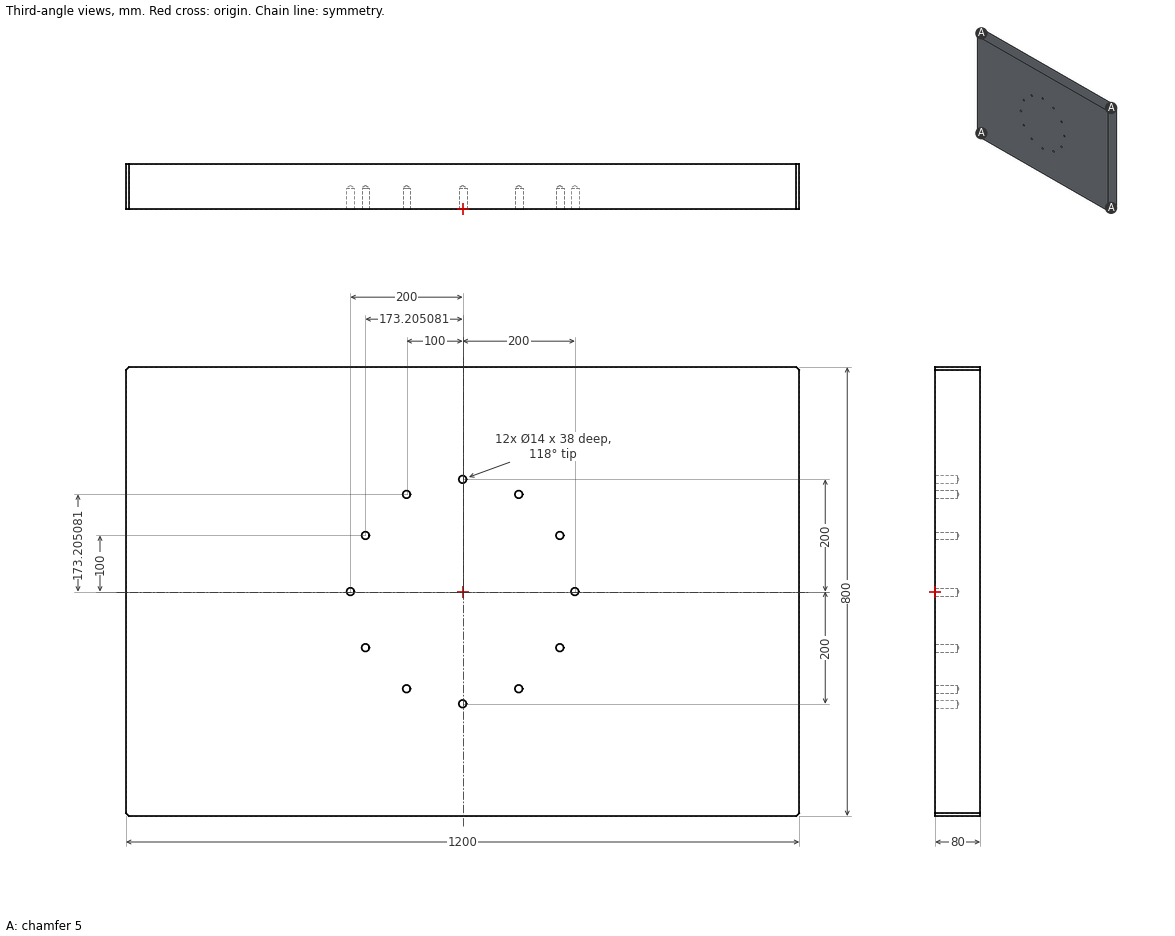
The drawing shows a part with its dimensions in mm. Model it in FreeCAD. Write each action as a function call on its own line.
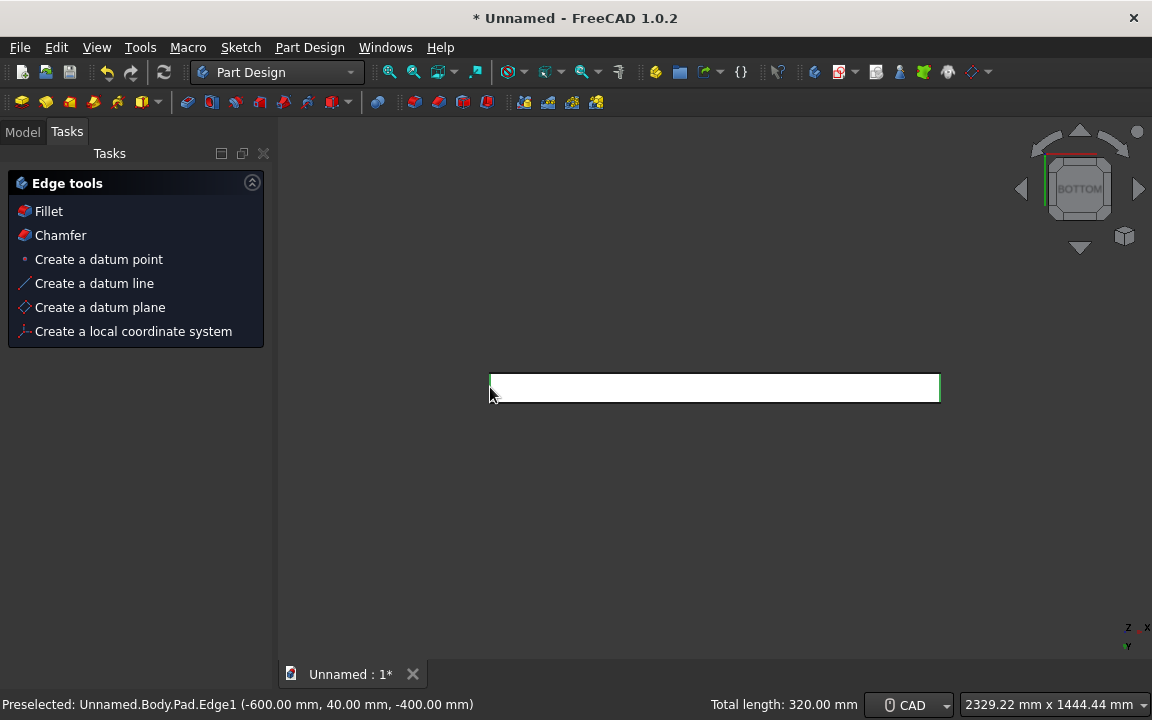
click(440, 102)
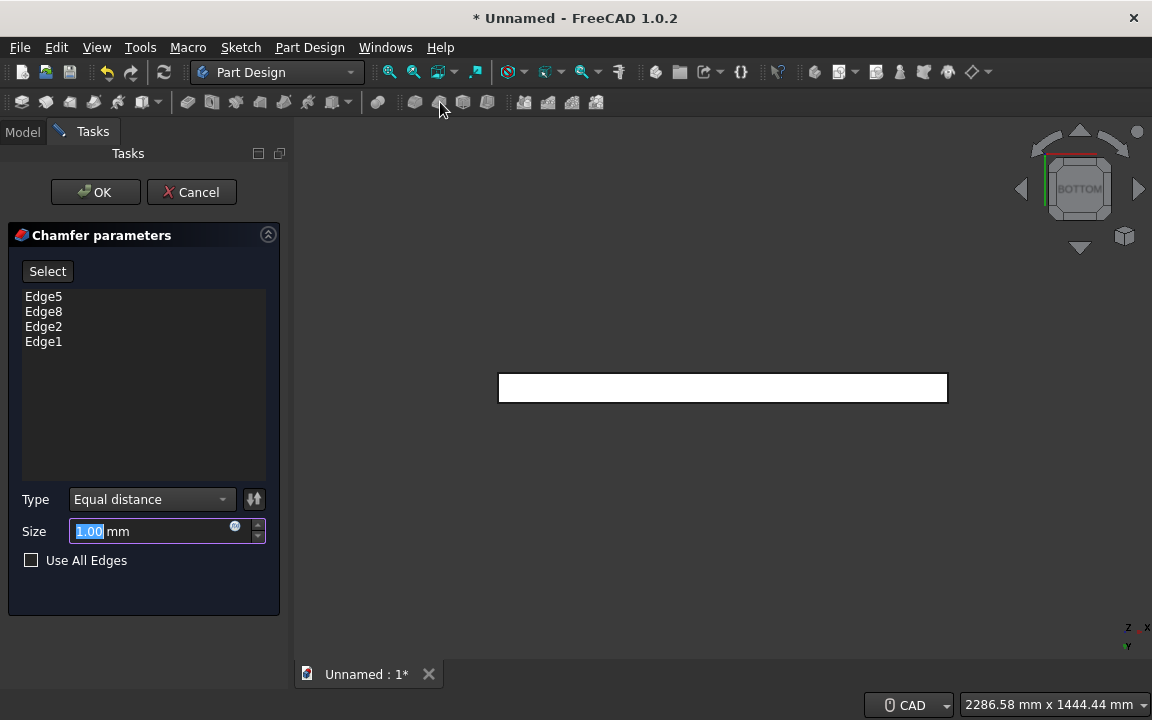
text(5)
key(Tab)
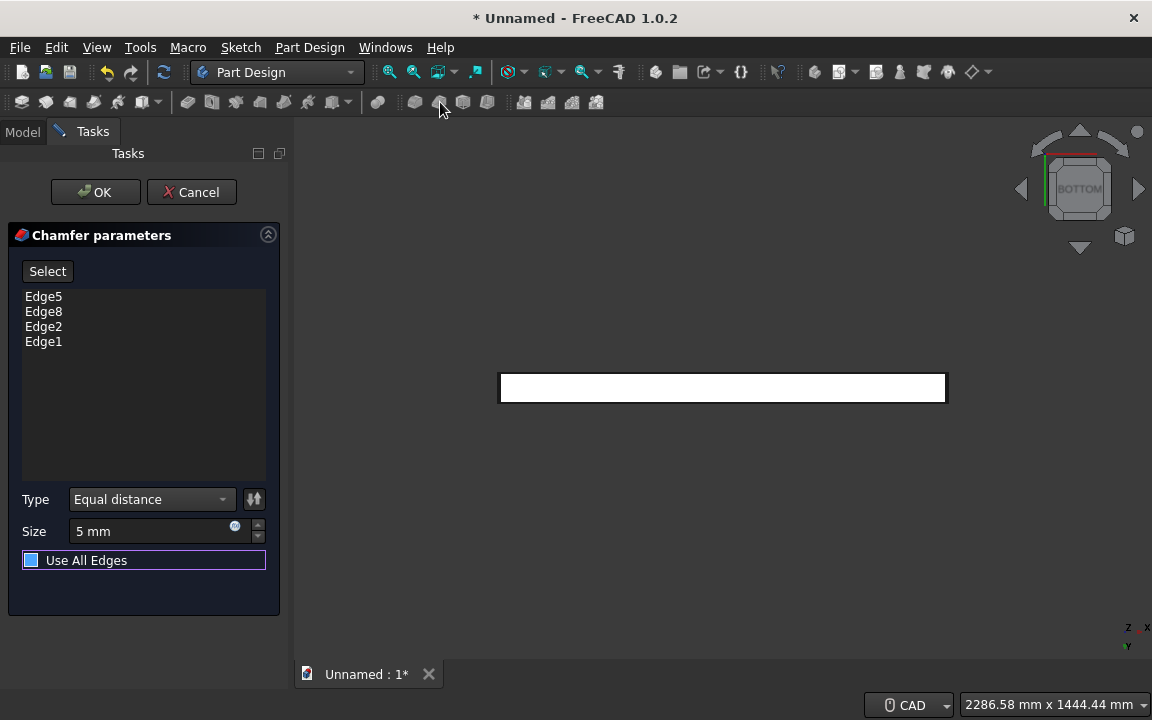
click(96, 192)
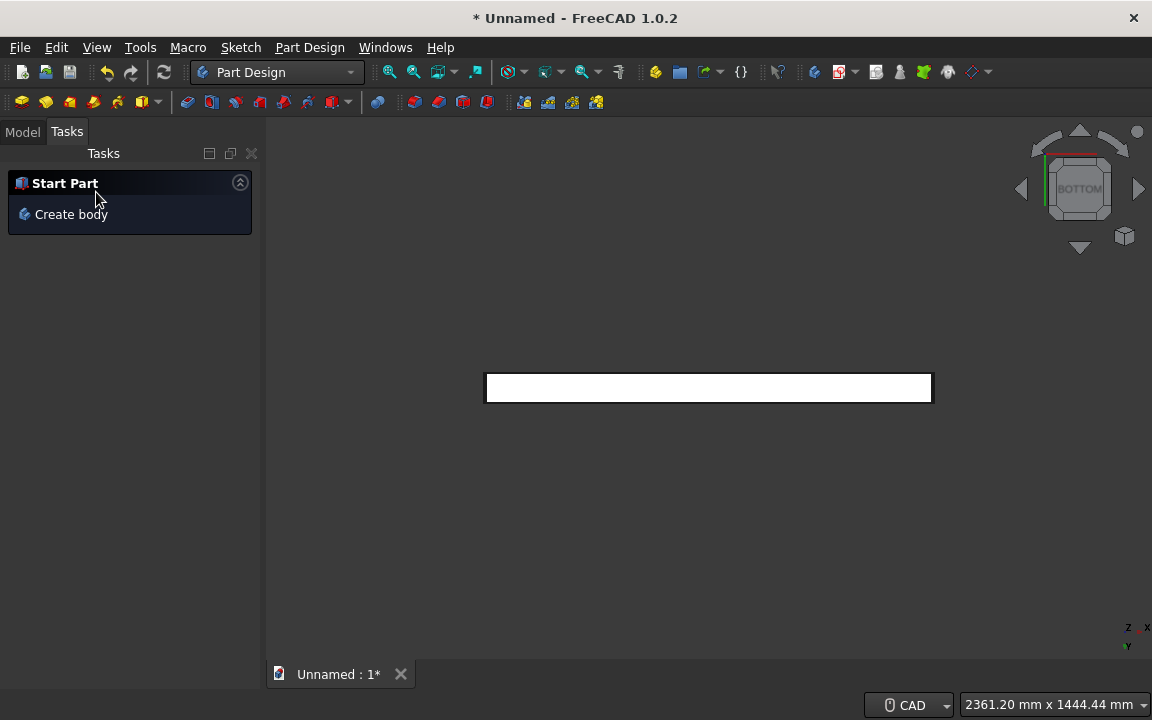
click(840, 72)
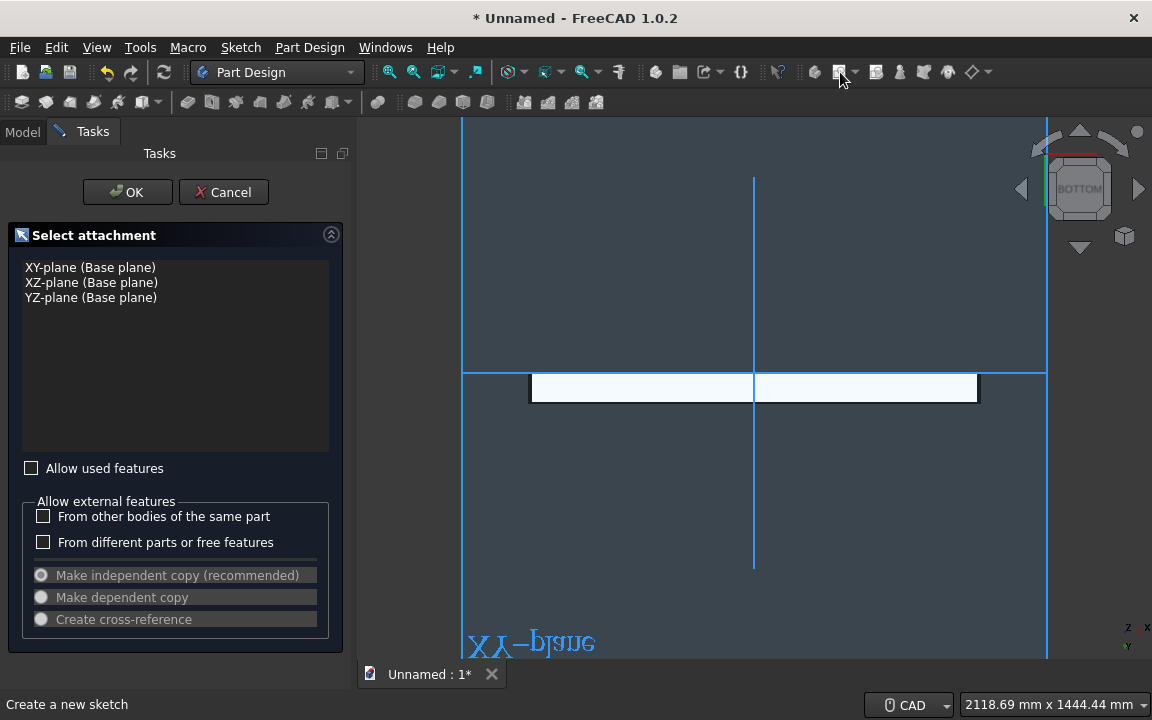
click(82, 282)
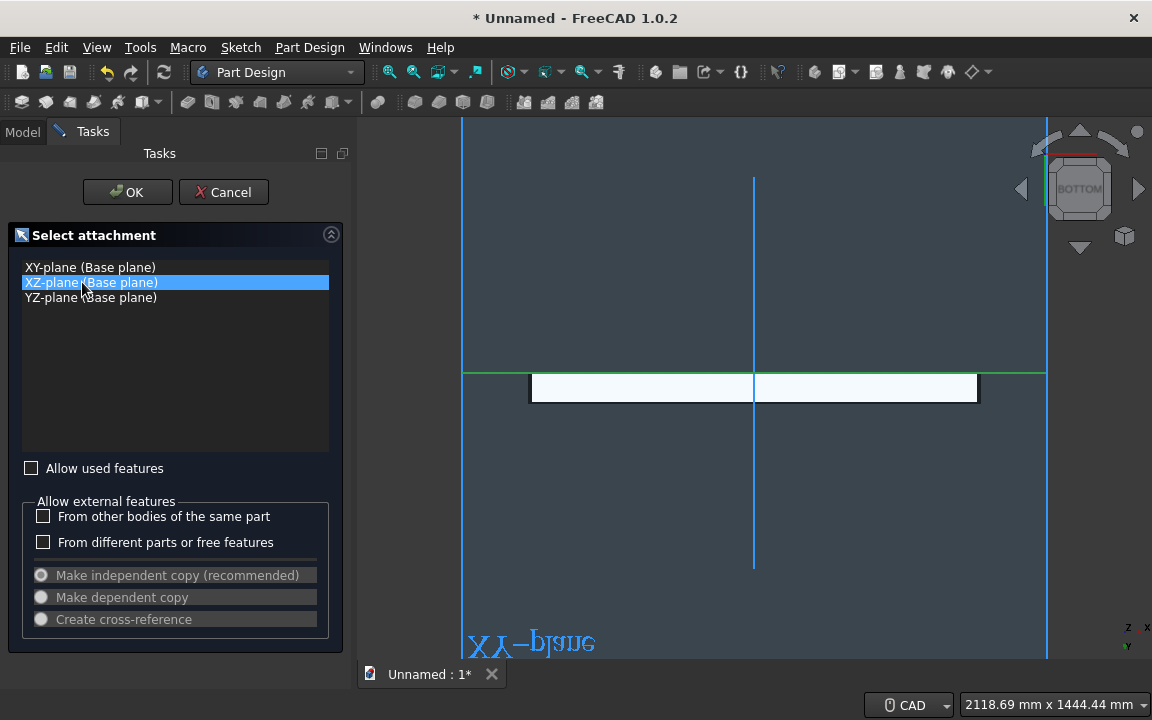
click(128, 192)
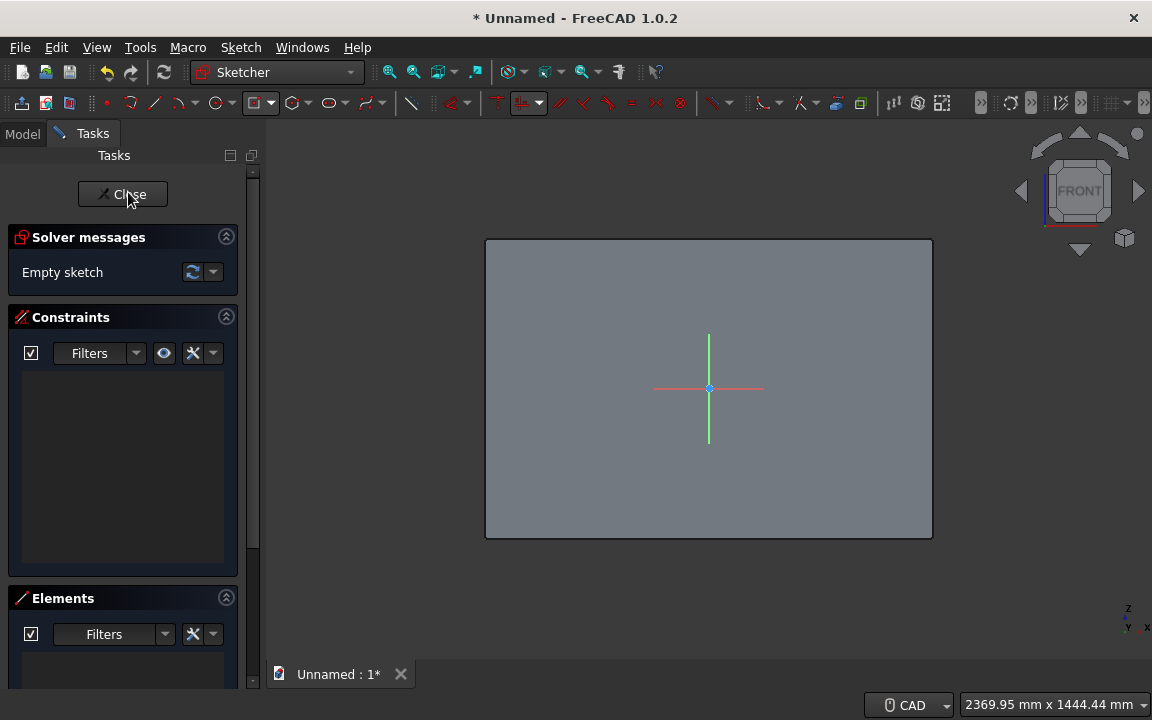
scroll(765, 389, up, 4)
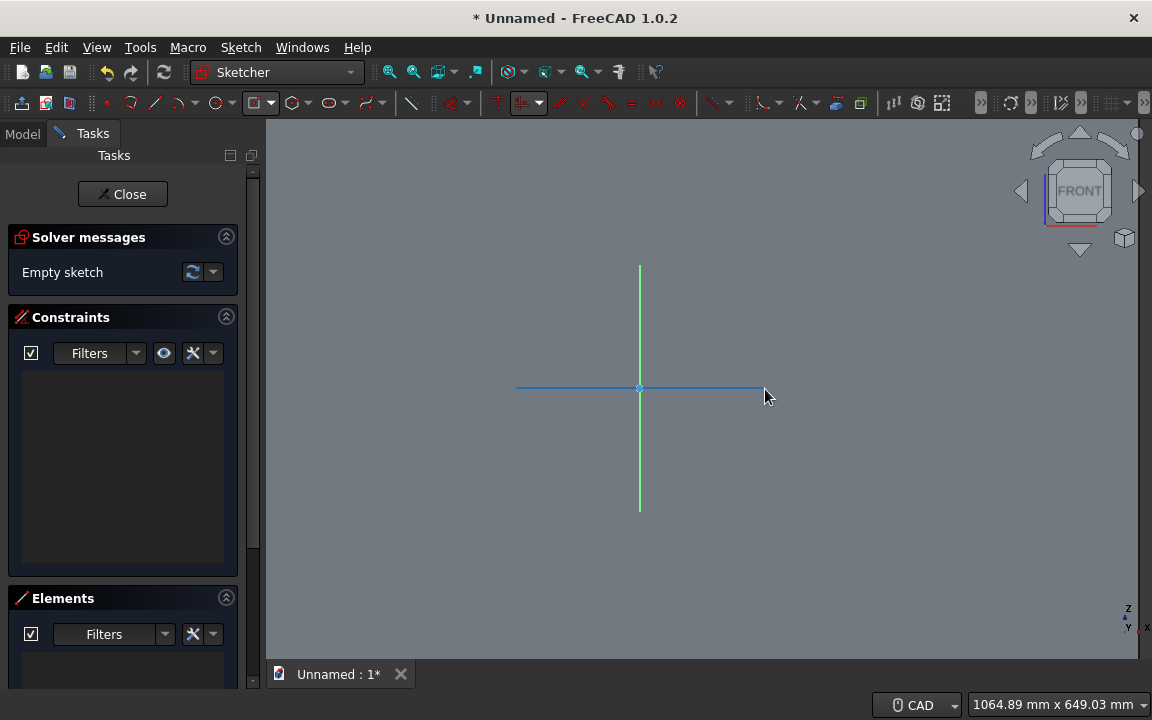
click(216, 104)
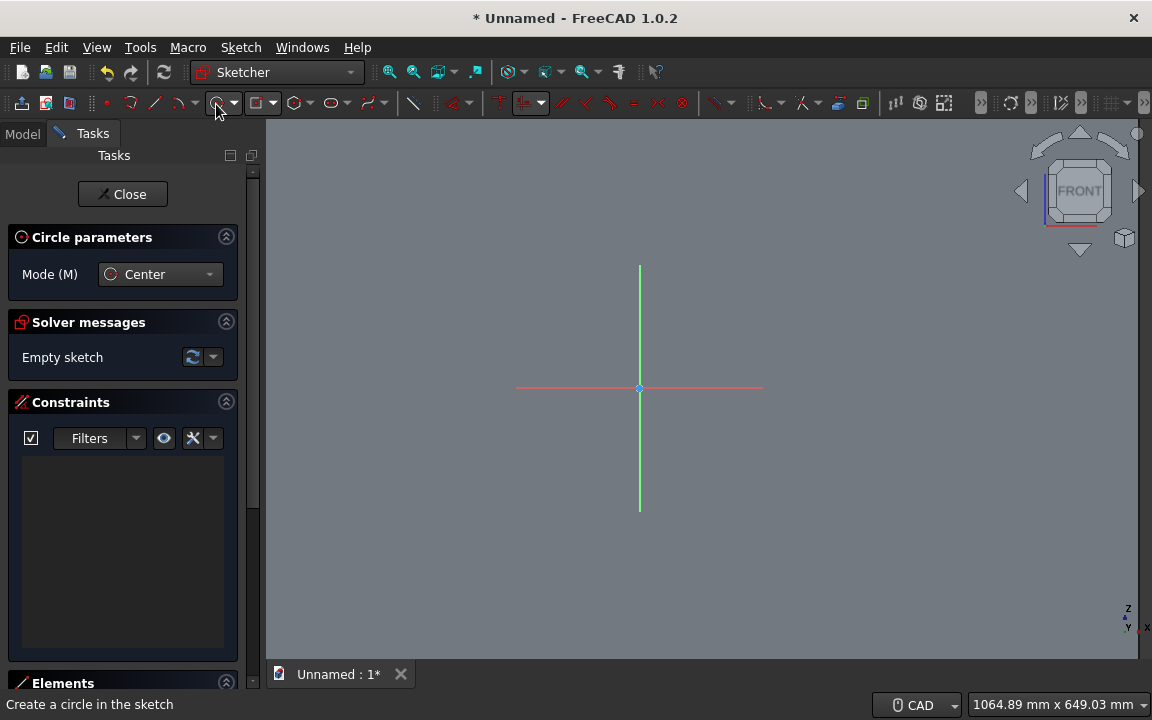
scroll(640, 222, up, 7)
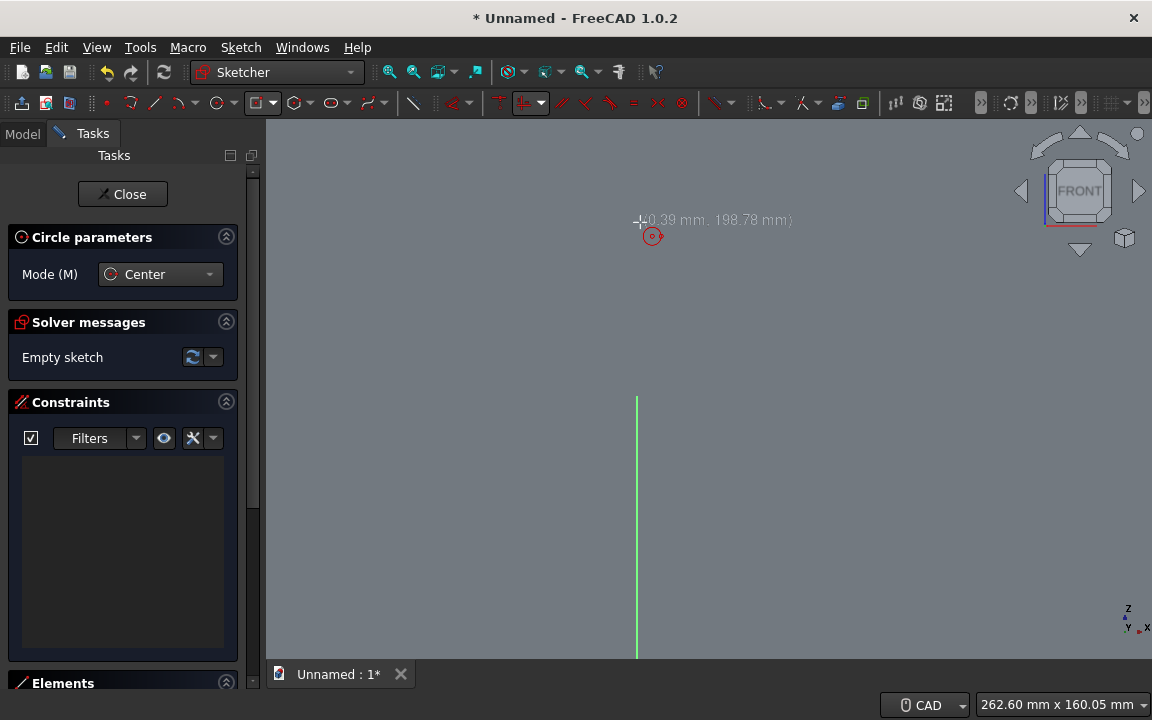
scroll(642, 223, down, 7)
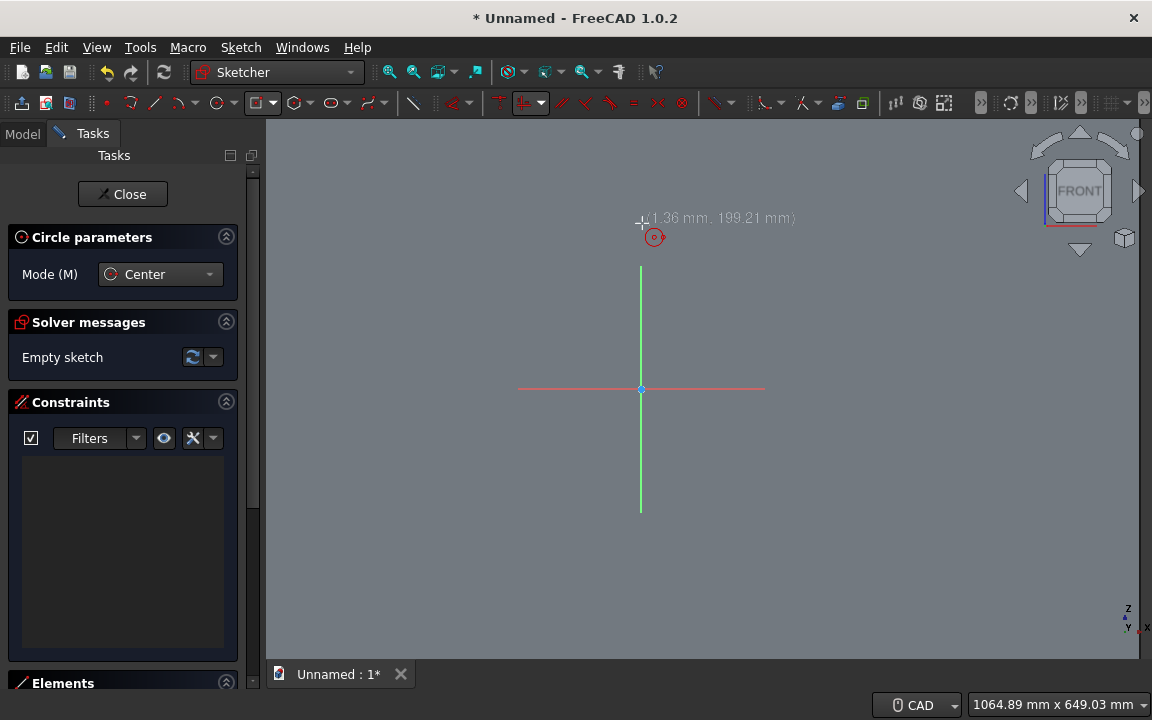
click(641, 223)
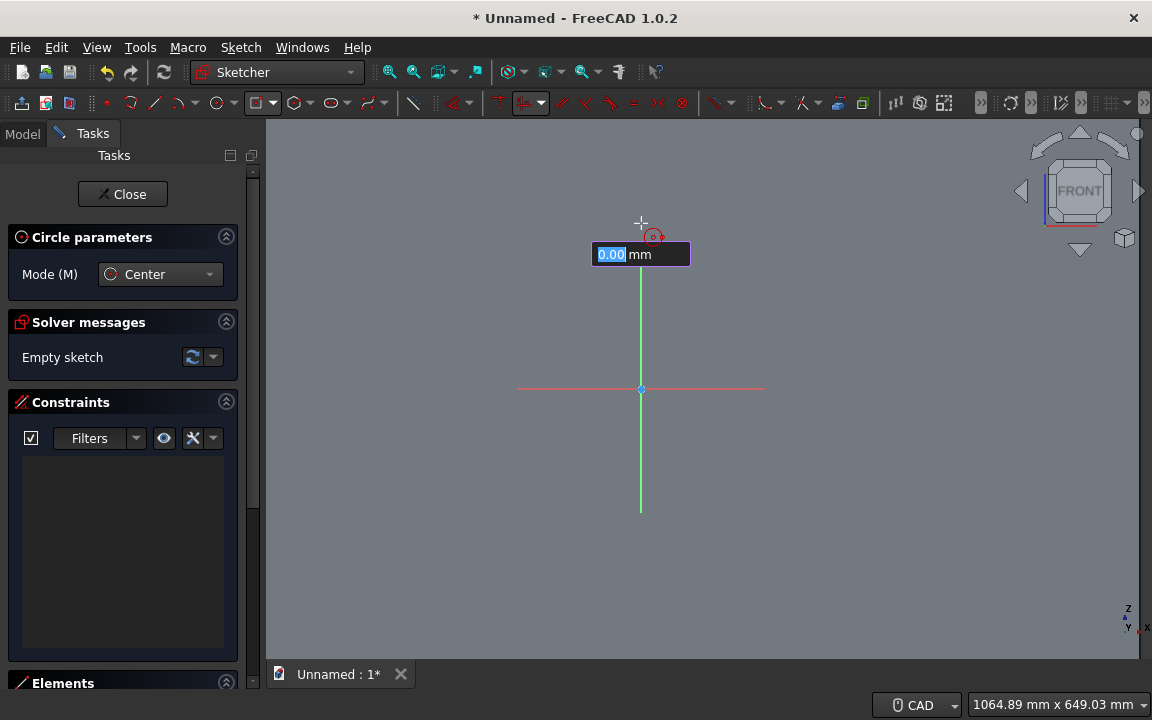
scroll(647, 221, up, 6)
move(645, 220)